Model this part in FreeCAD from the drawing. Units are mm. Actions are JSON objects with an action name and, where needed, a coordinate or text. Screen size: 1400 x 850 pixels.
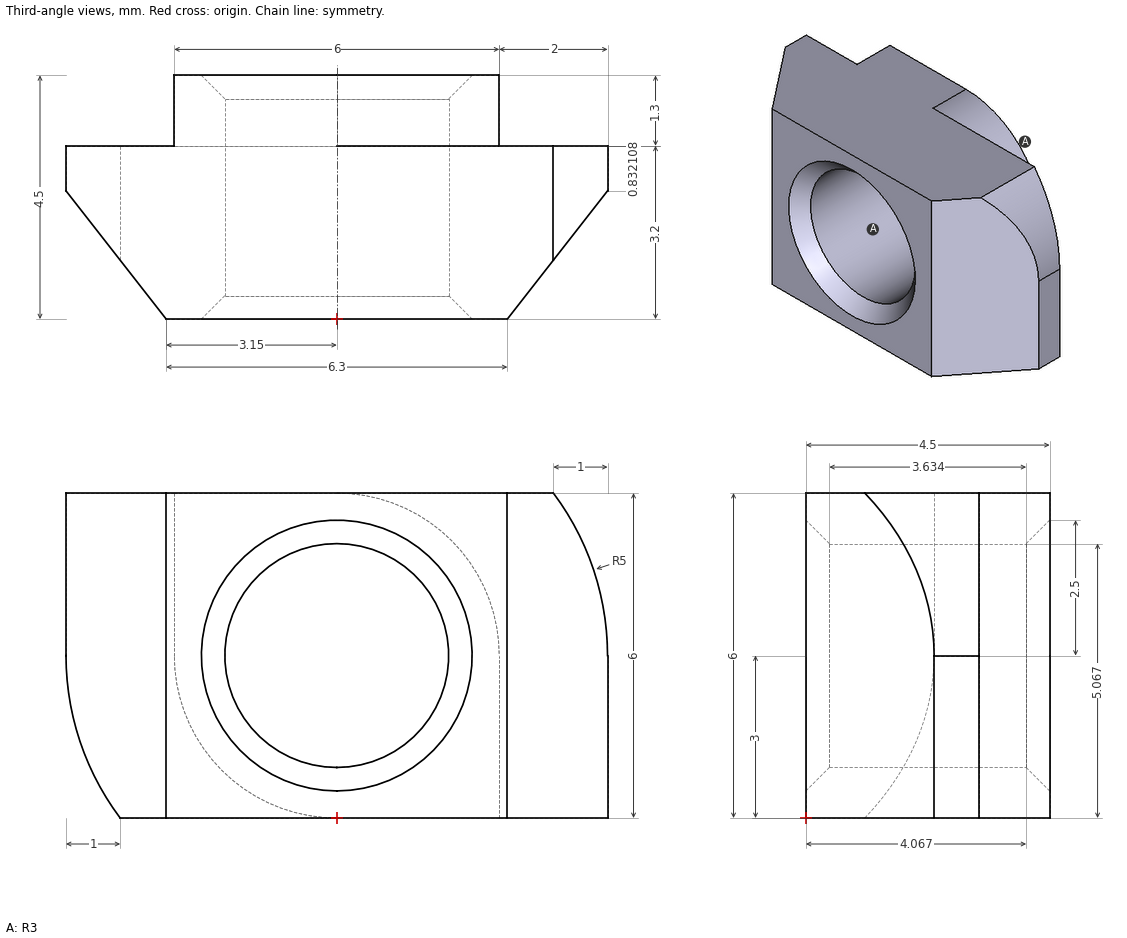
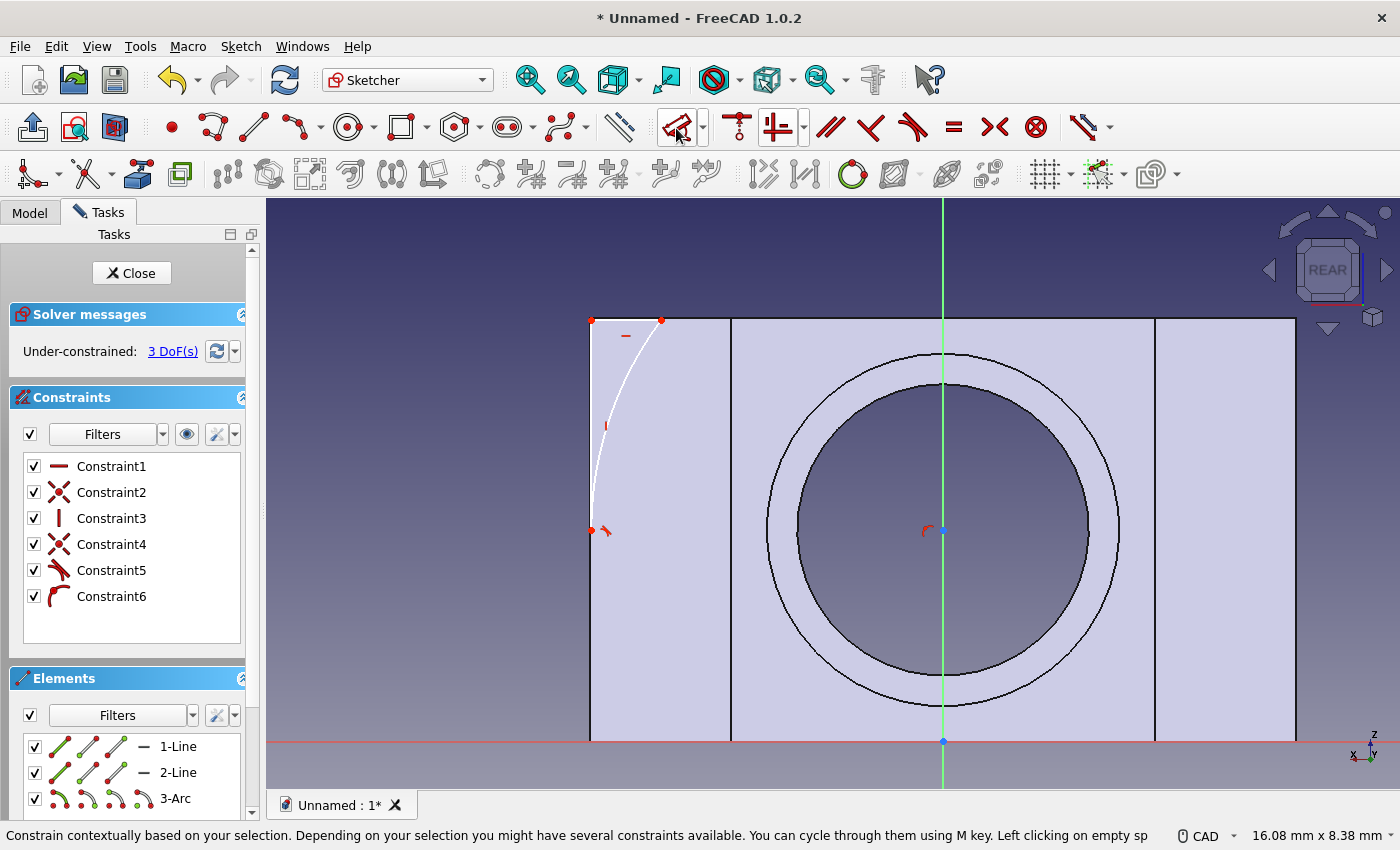
{"action": "left_click", "coordinate": [626, 378]}
{"action": "left_click", "coordinate": [560, 550]}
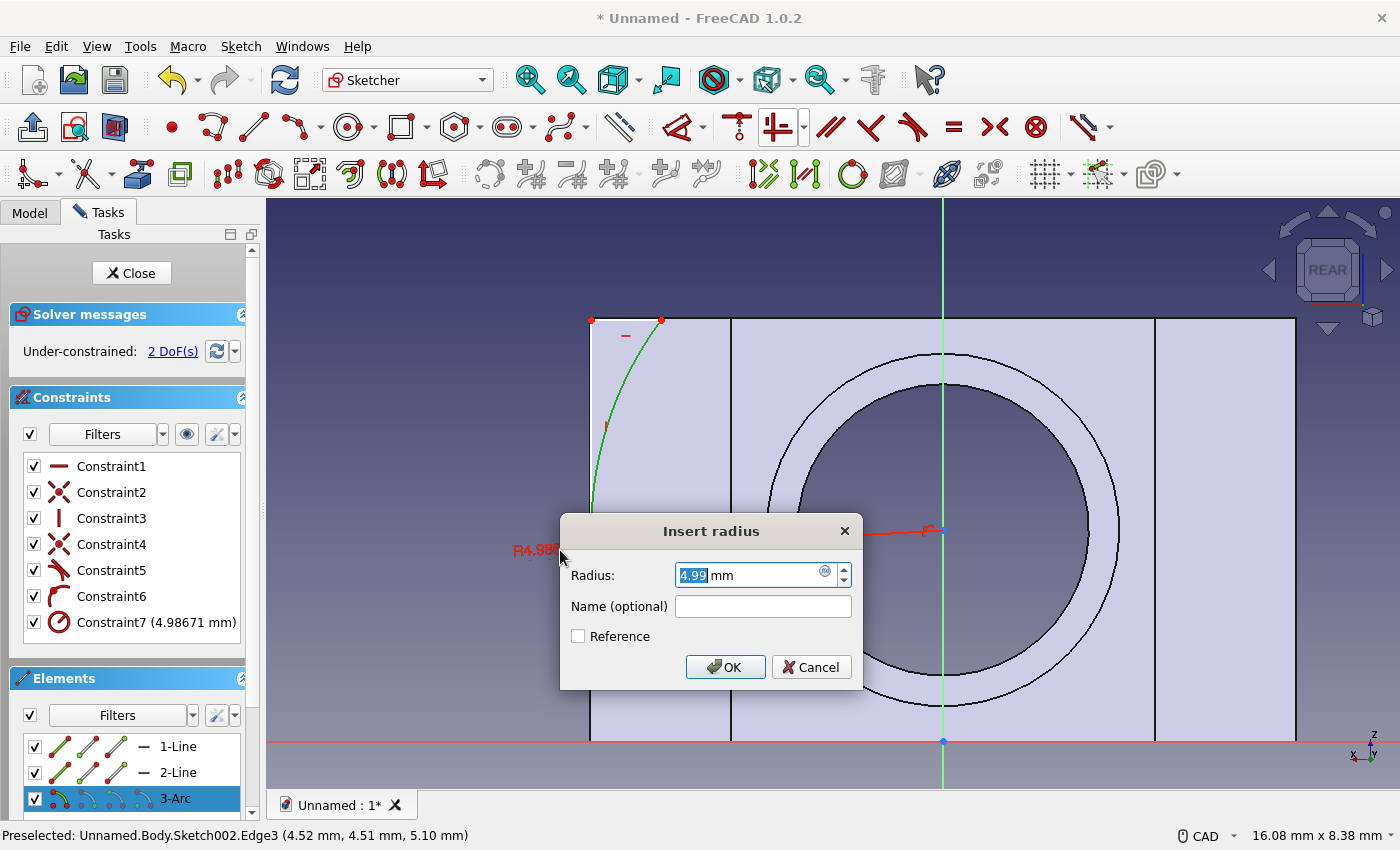
{"action": "type", "text": "5"}
{"action": "key", "text": "Return"}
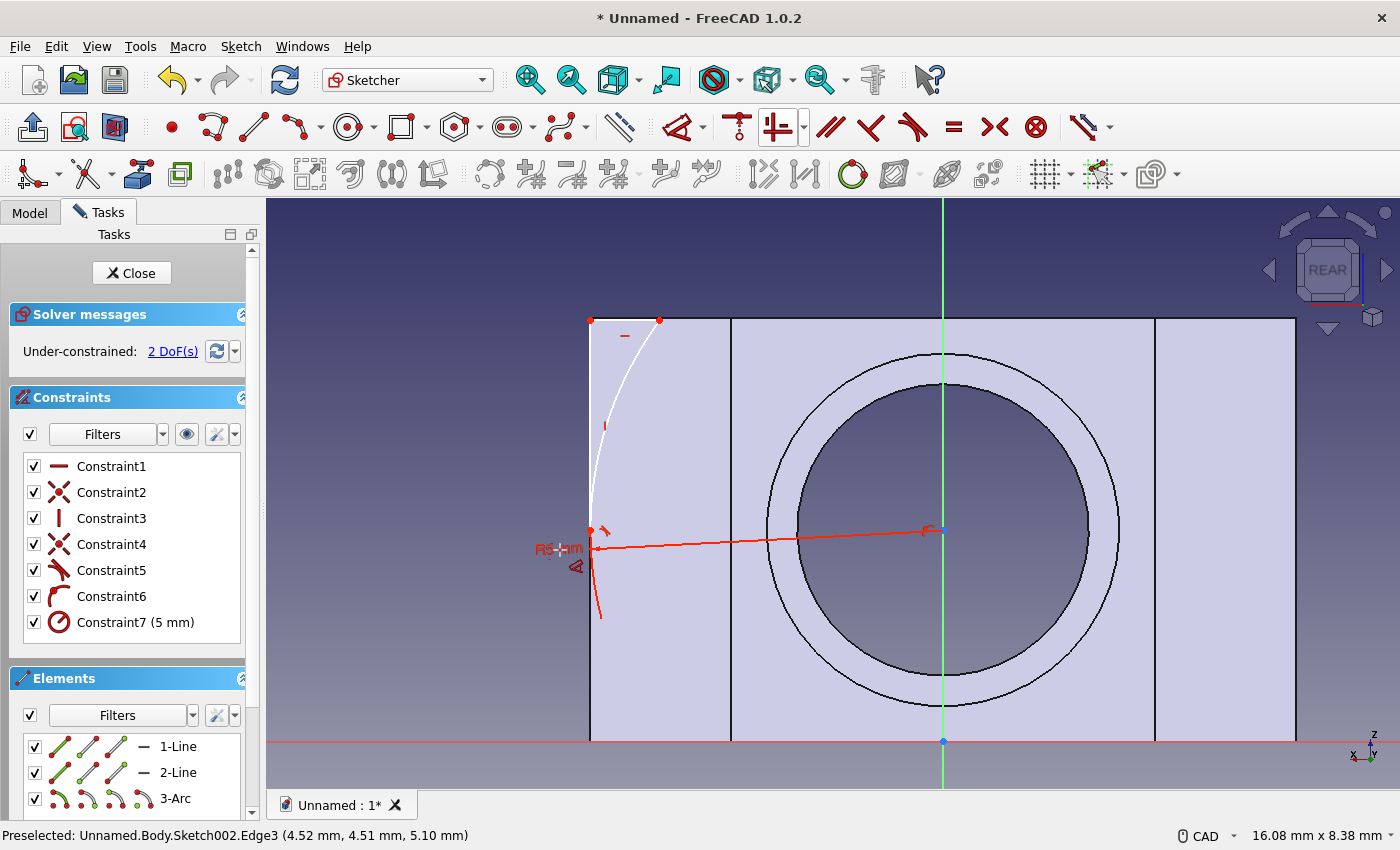
{"action": "left_click", "coordinate": [639, 320]}
{"action": "left_click", "coordinate": [625, 286]}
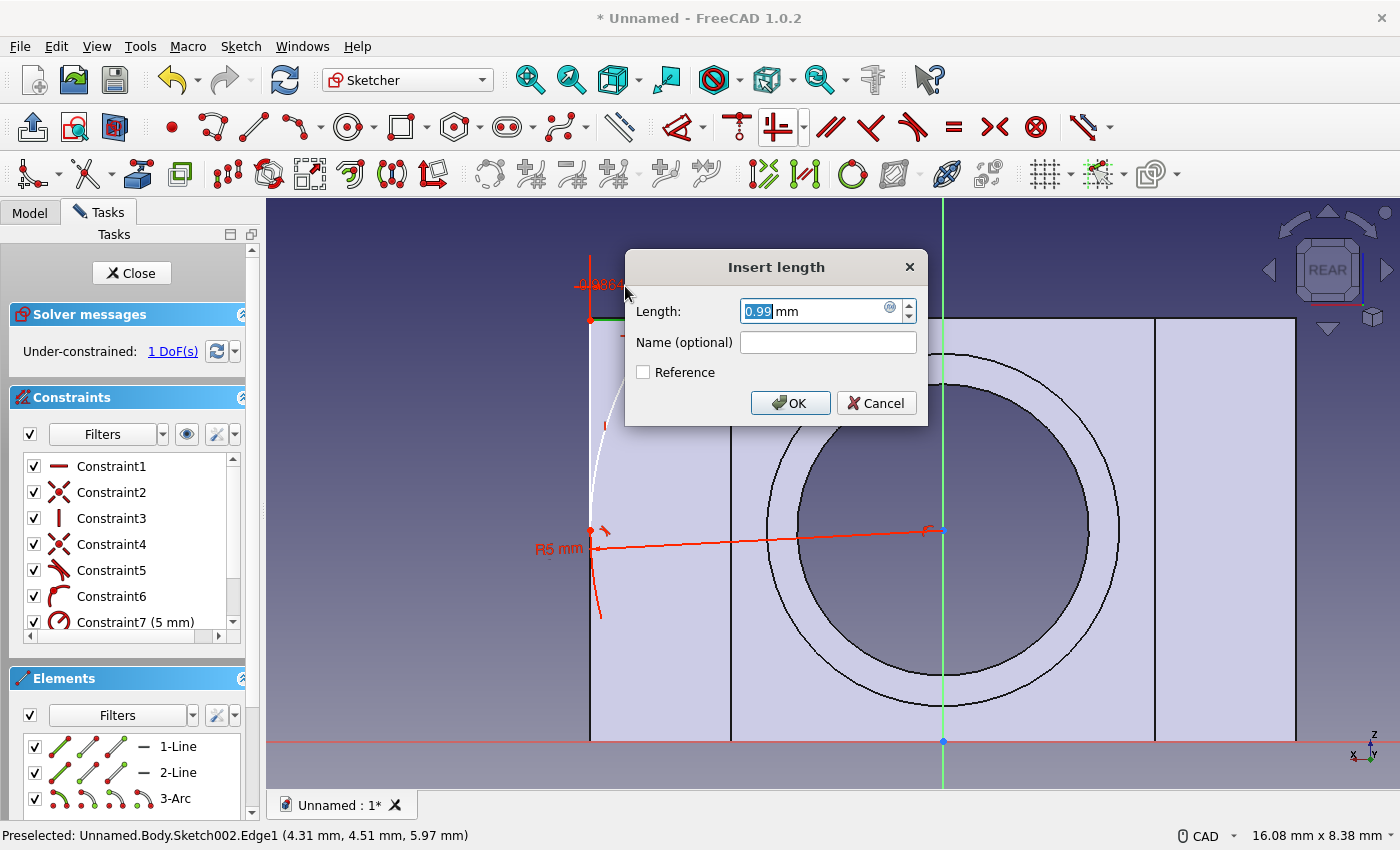
{"action": "type", "text": "1"}
{"action": "key", "text": "Return"}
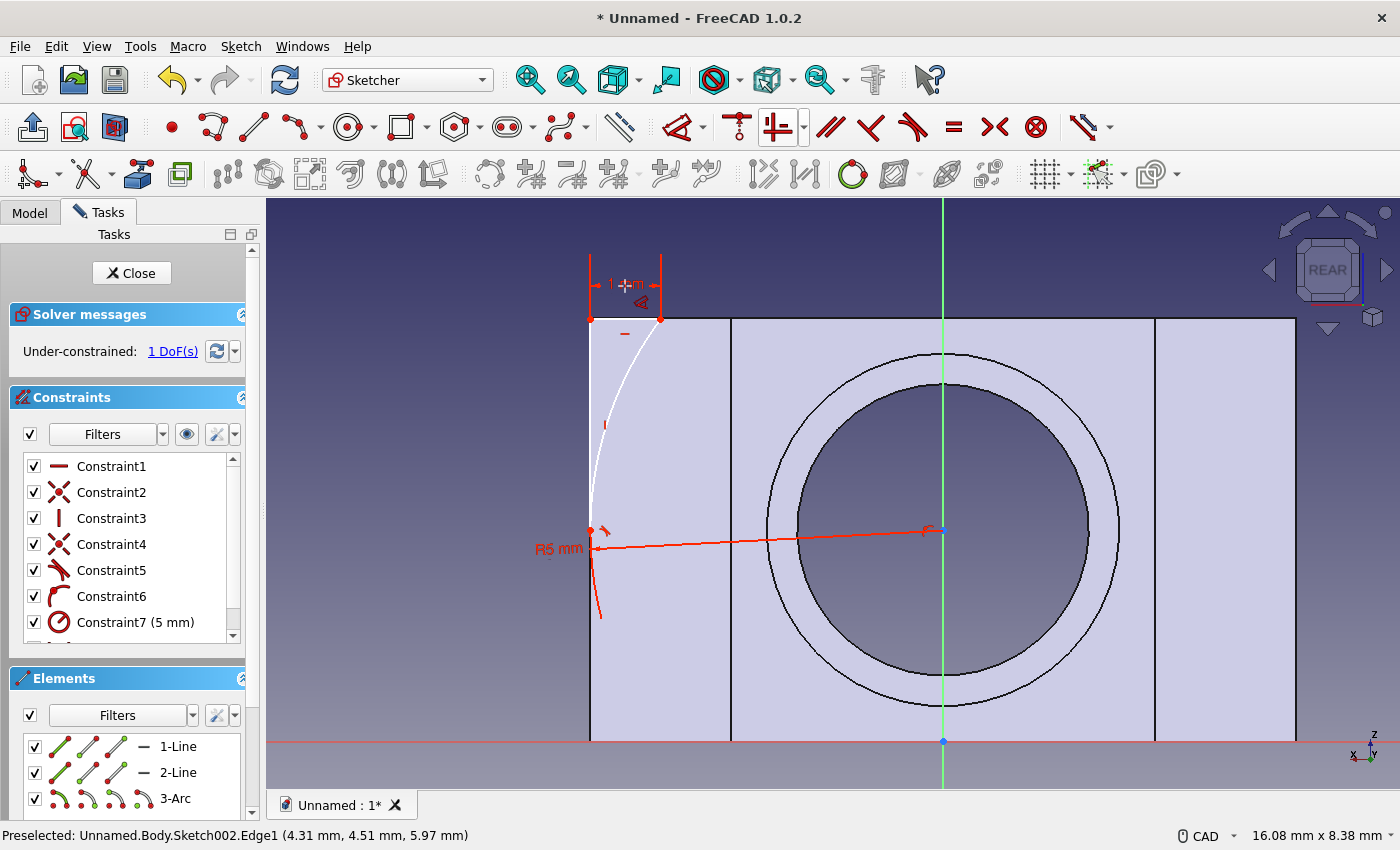
{"action": "left_click", "coordinate": [661, 319]}
{"action": "left_click", "coordinate": [977, 530]}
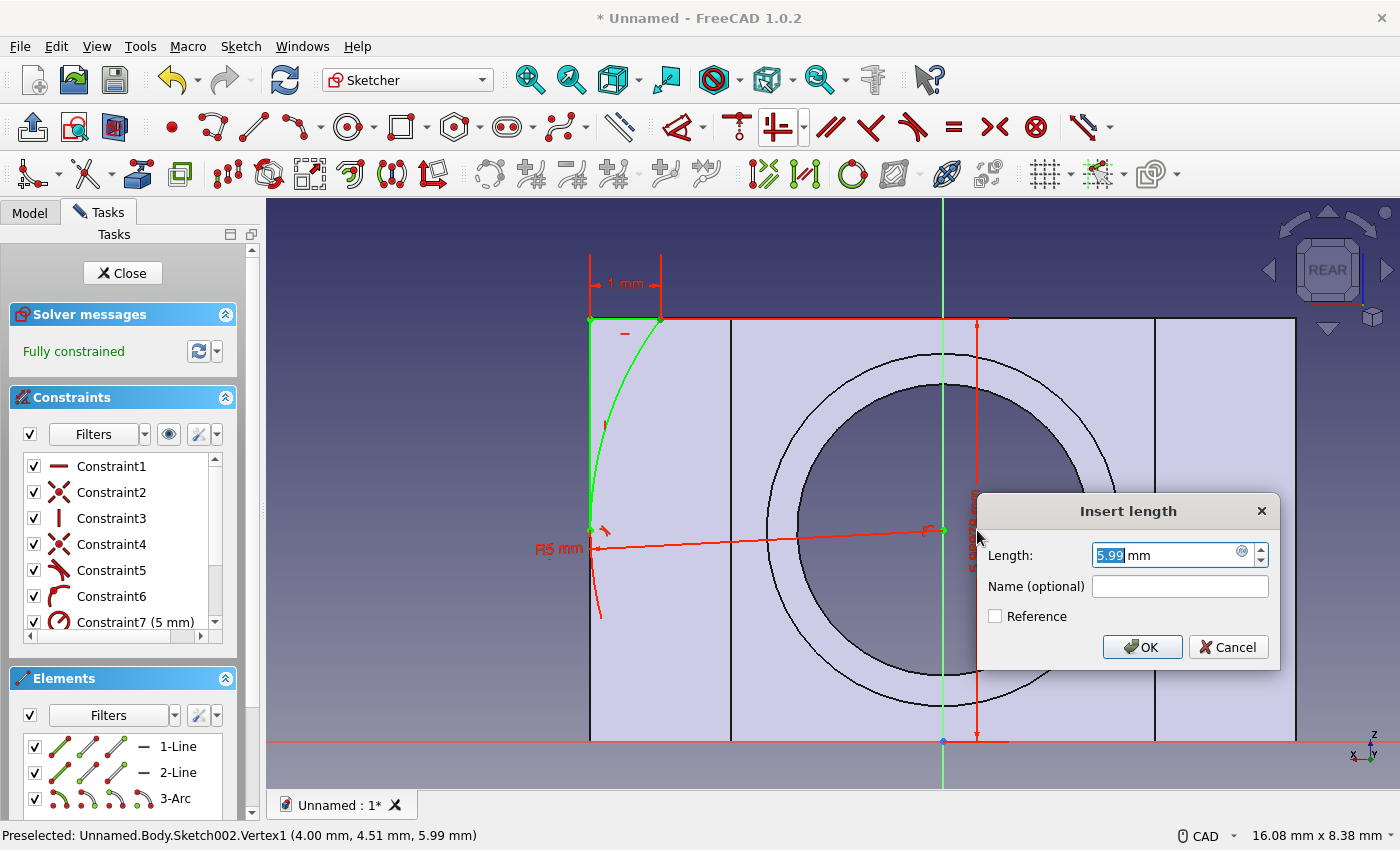
{"action": "type", "text": "6"}
{"action": "key", "text": "Return"}
{"action": "key", "text": "Escape"}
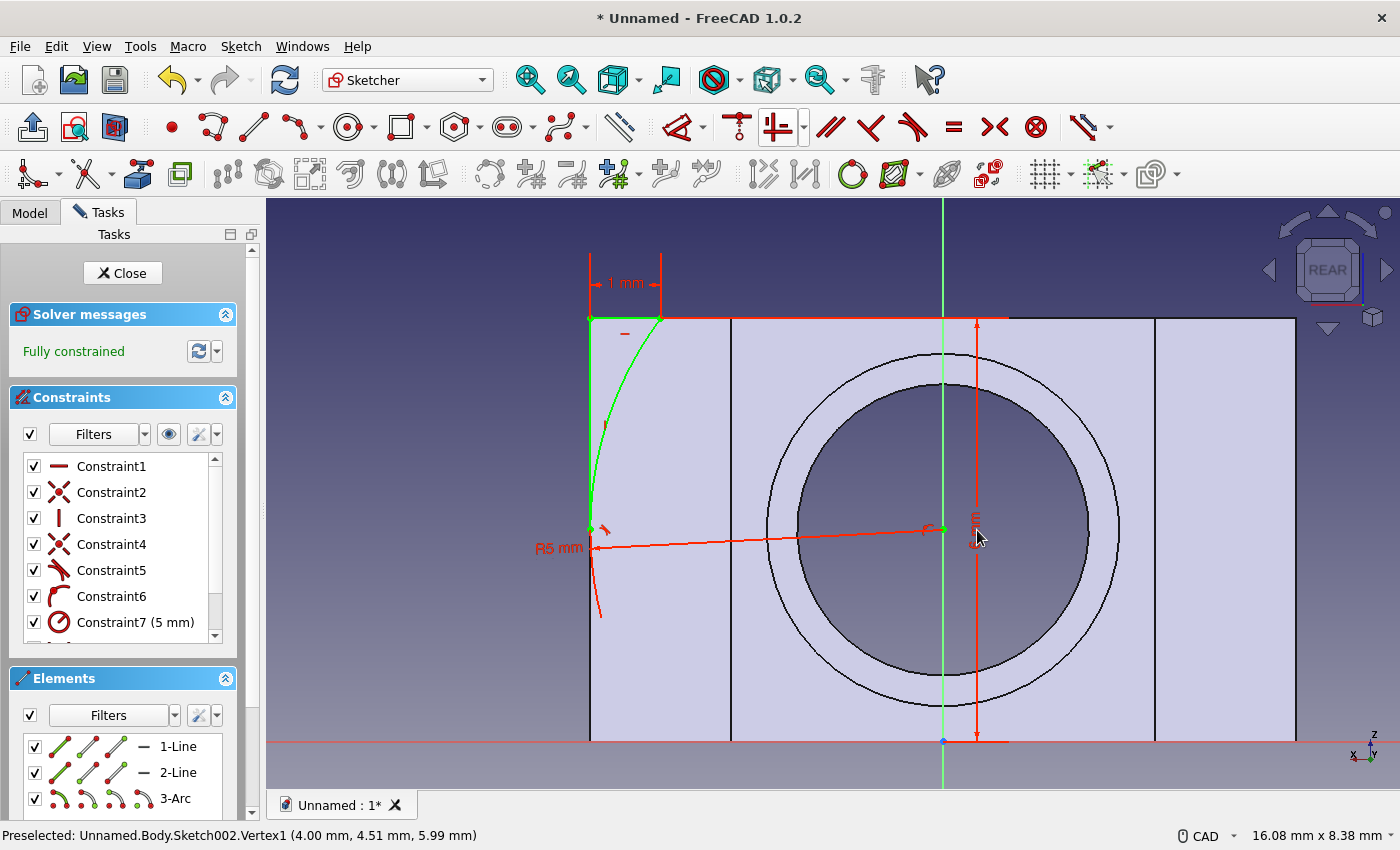
{"action": "left_click", "coordinate": [123, 273]}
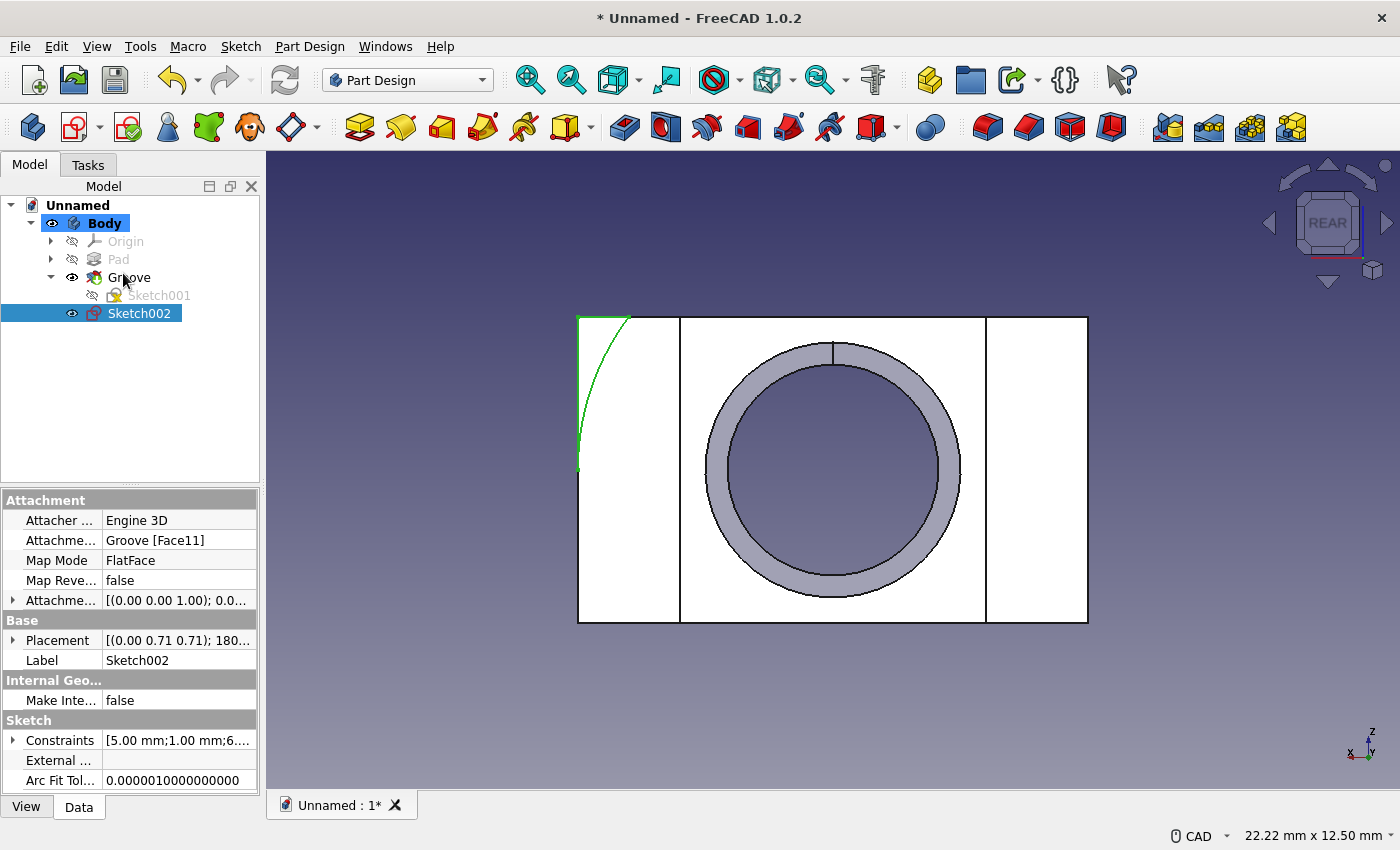
{"action": "left_click", "coordinate": [625, 128]}